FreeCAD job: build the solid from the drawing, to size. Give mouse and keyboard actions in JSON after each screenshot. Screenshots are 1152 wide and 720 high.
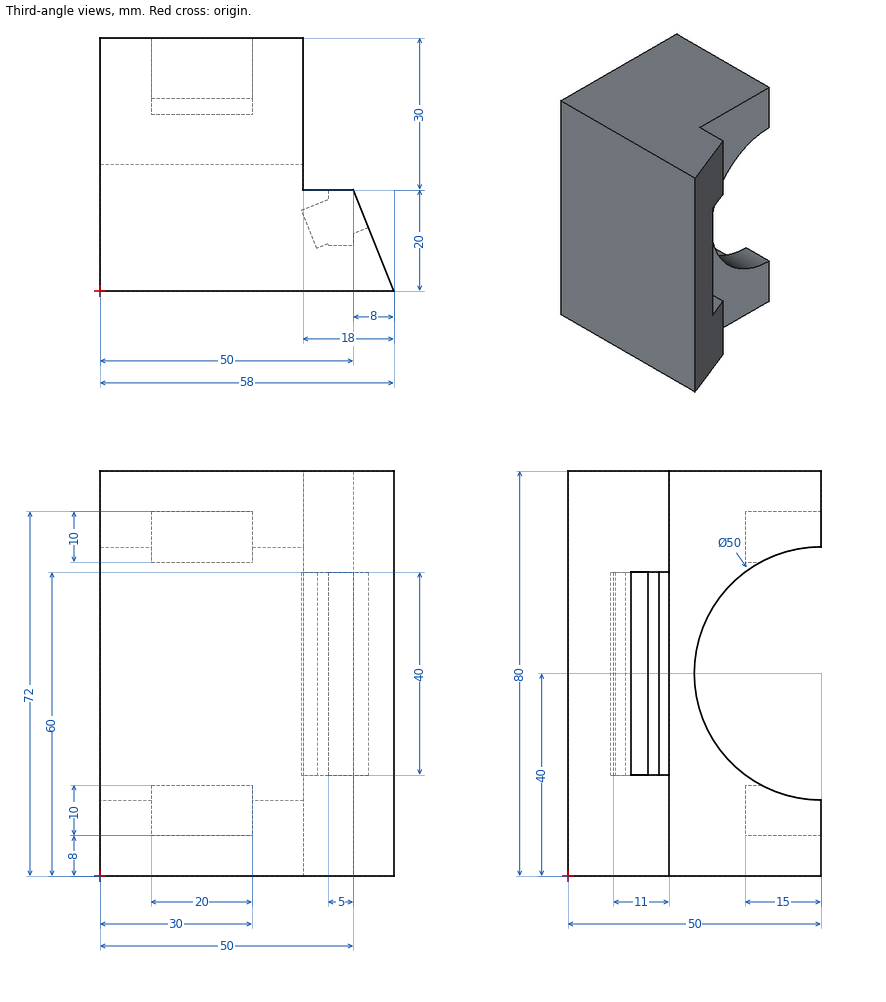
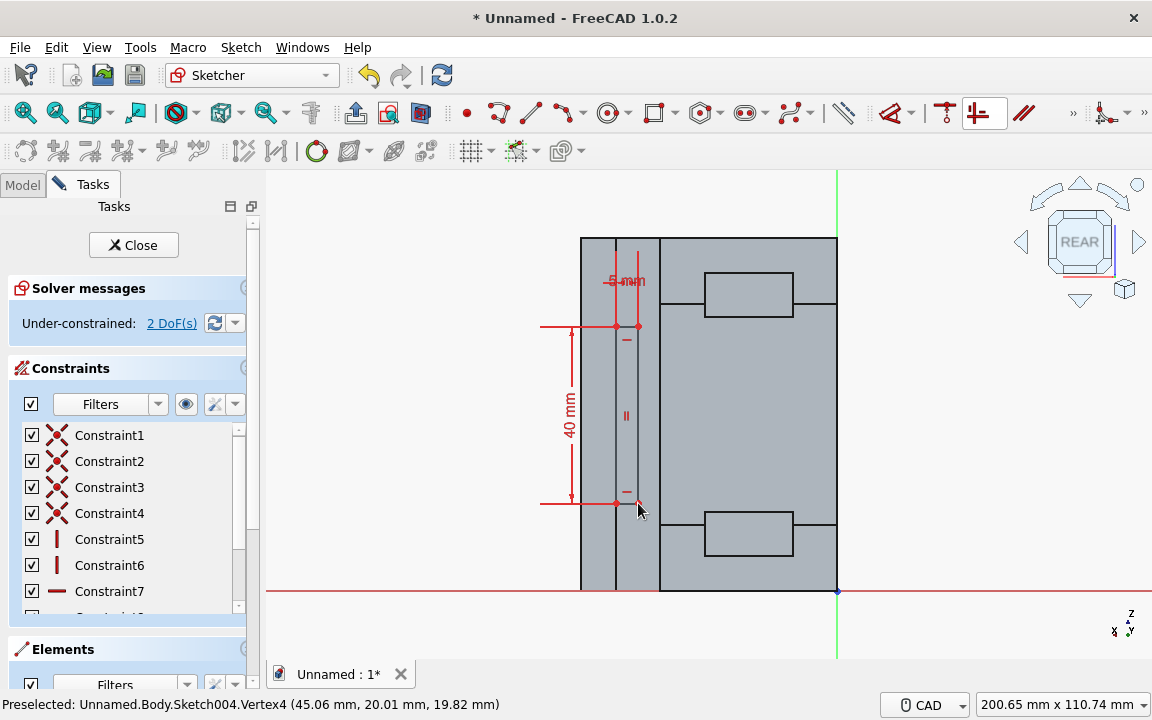
{"action": "left_click", "coordinate": [890, 114]}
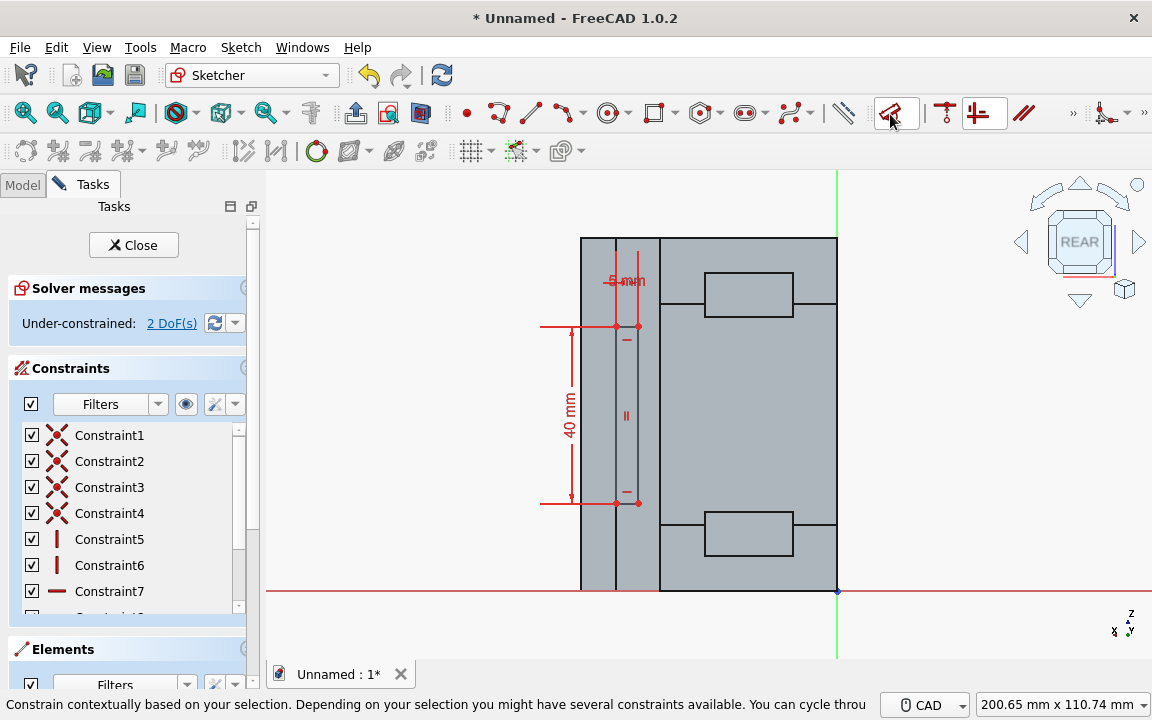
{"action": "left_click", "coordinate": [616, 327]}
{"action": "left_click", "coordinate": [727, 625]}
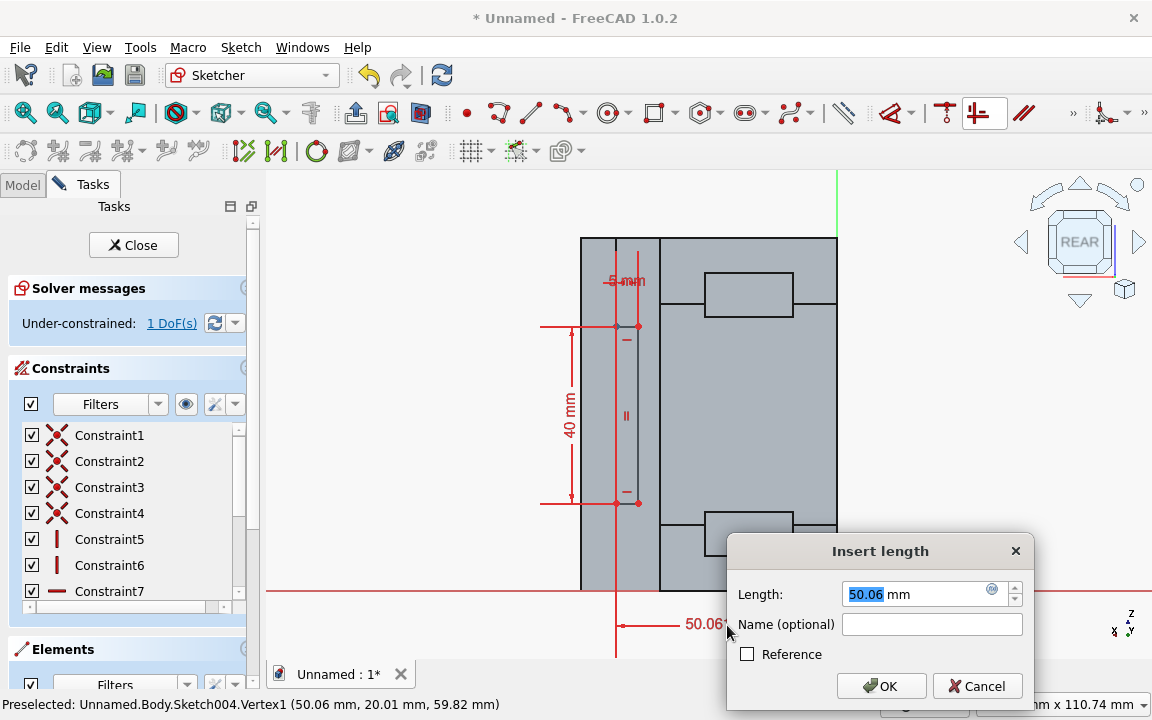
{"action": "type", "text": "50"}
{"action": "key", "text": "Return"}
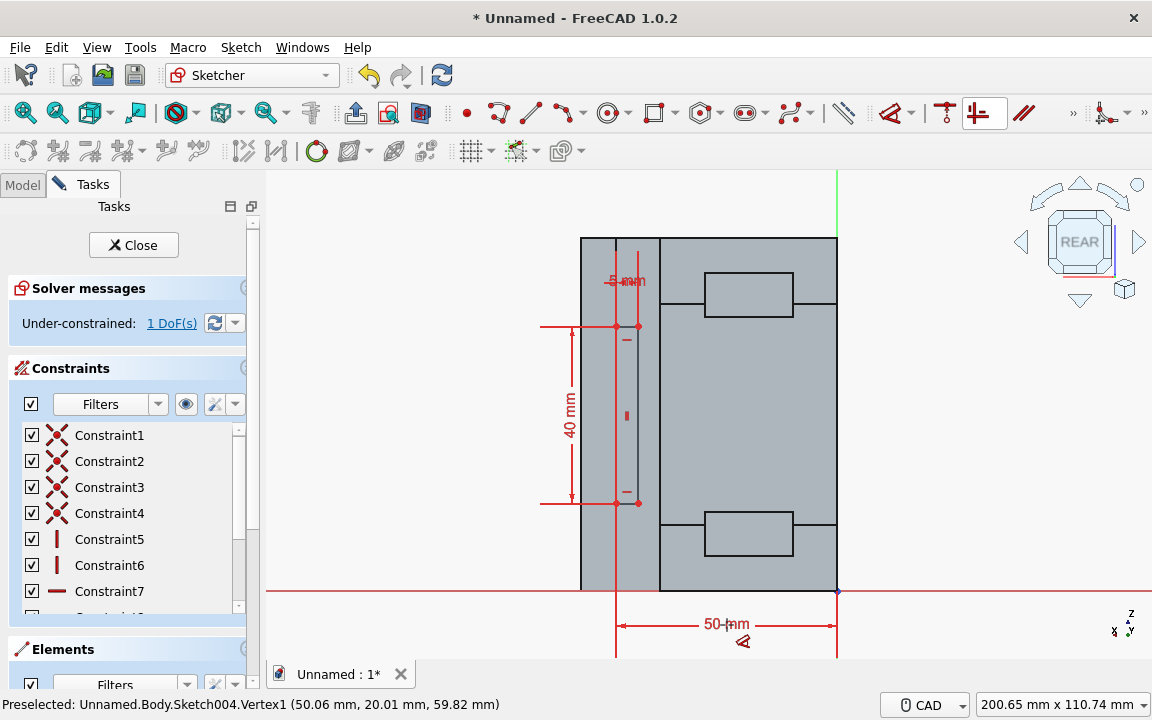
{"action": "left_click", "coordinate": [616, 327]}
{"action": "left_click", "coordinate": [871, 459]}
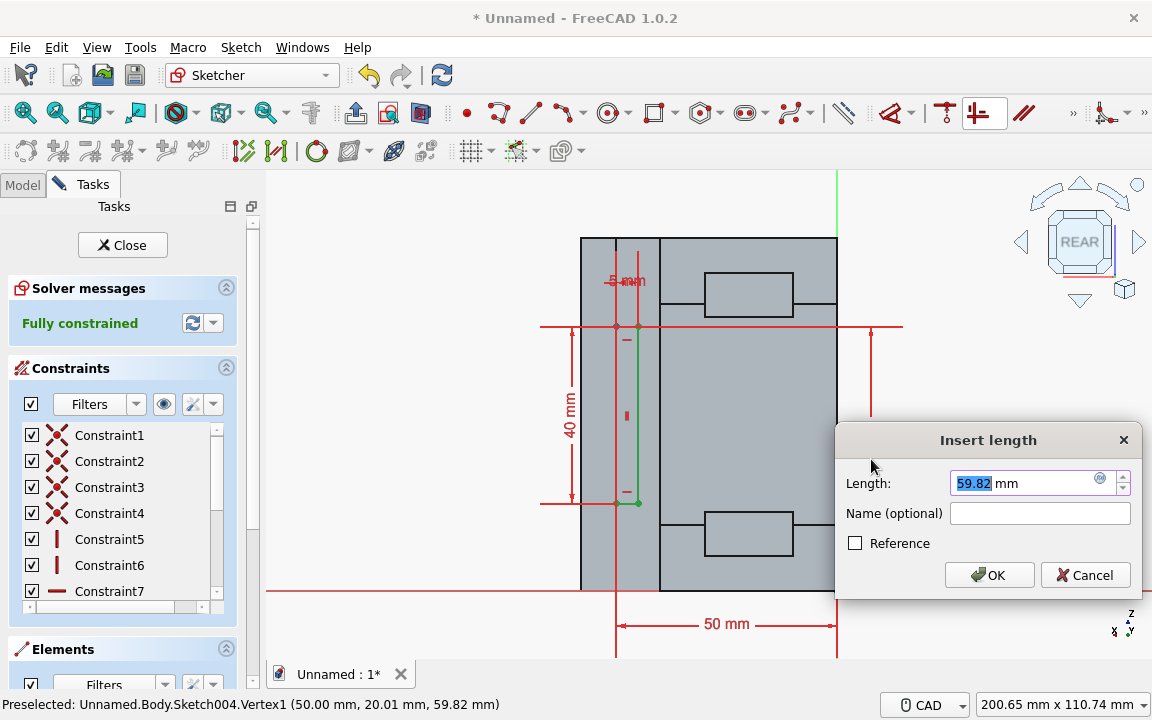
{"action": "type", "text": "60"}
{"action": "key", "text": "Return"}
{"action": "key", "text": "Escape"}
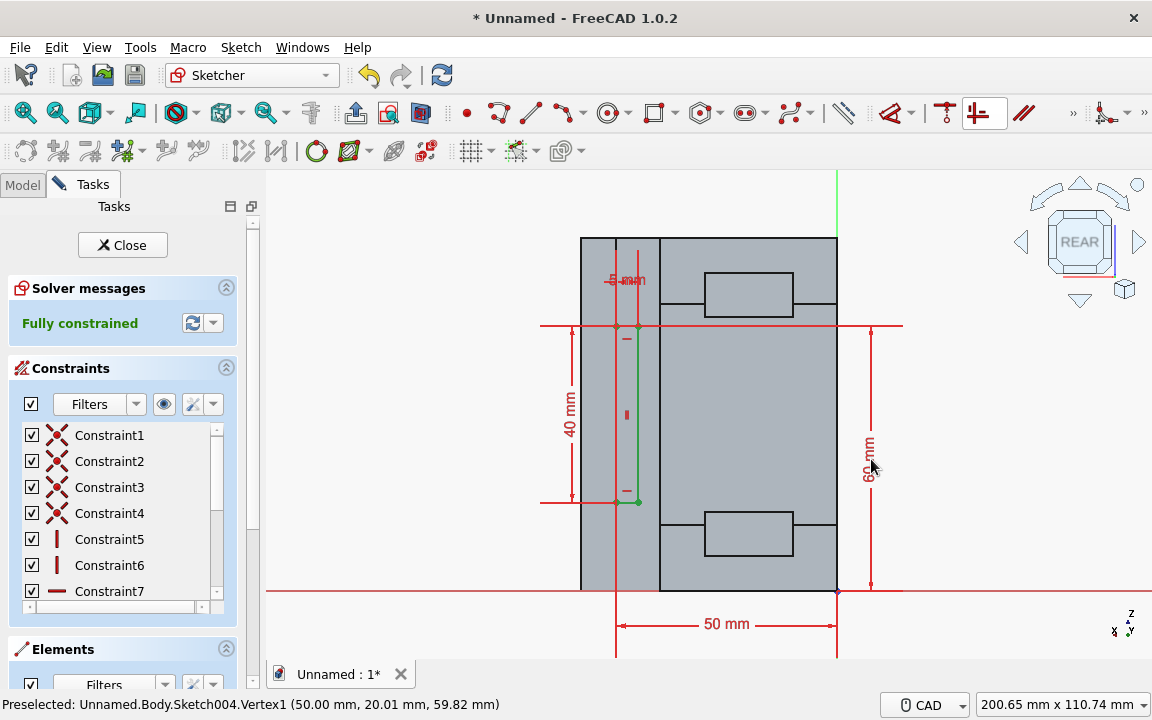
{"action": "left_click", "coordinate": [123, 245]}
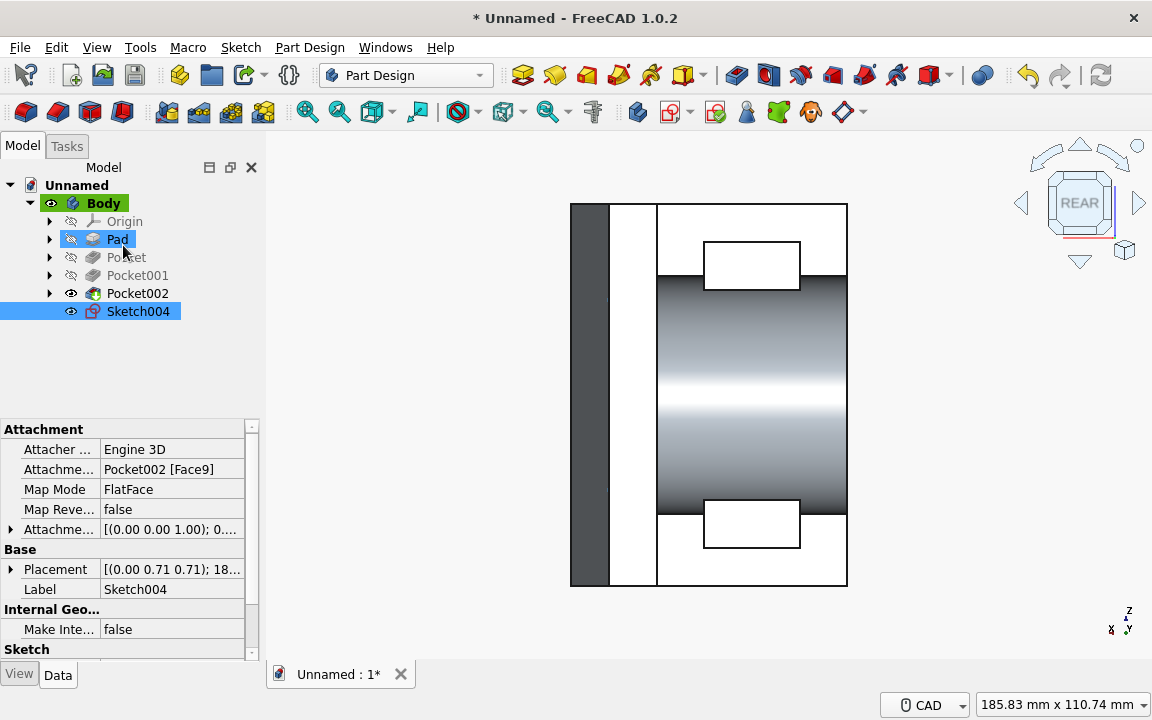
{"action": "left_click", "coordinate": [738, 76]}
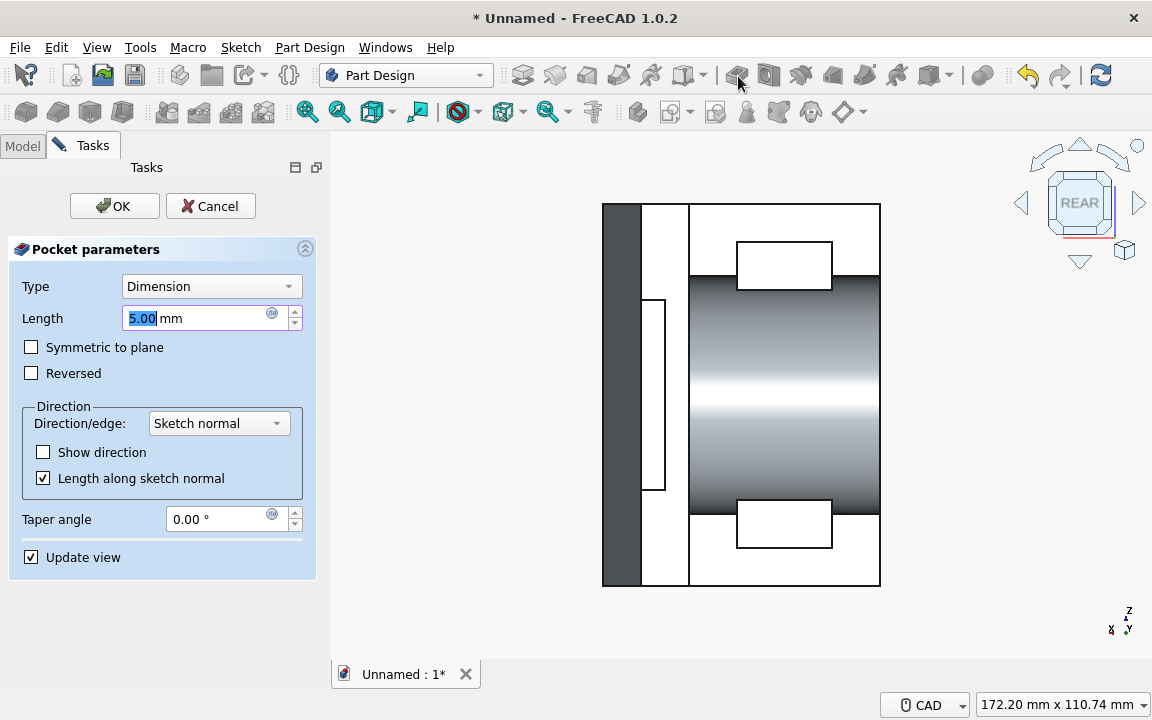
{"action": "type", "text": "11"}
{"action": "key", "text": "Tab"}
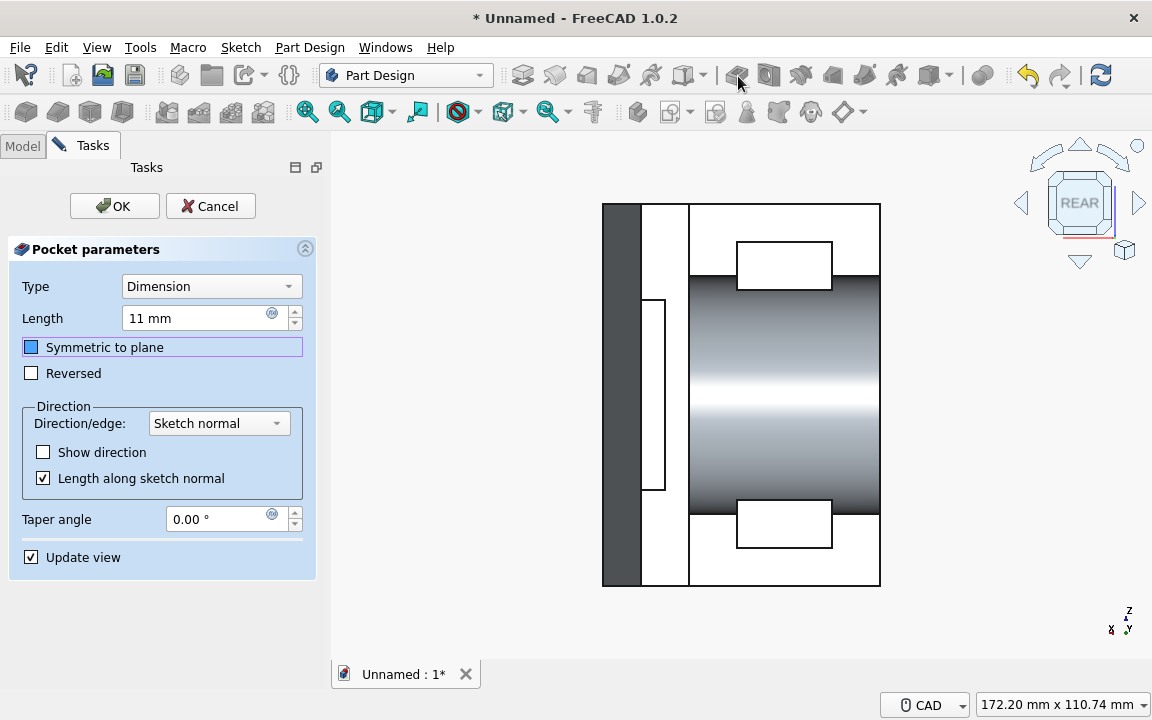
{"action": "left_click", "coordinate": [115, 206]}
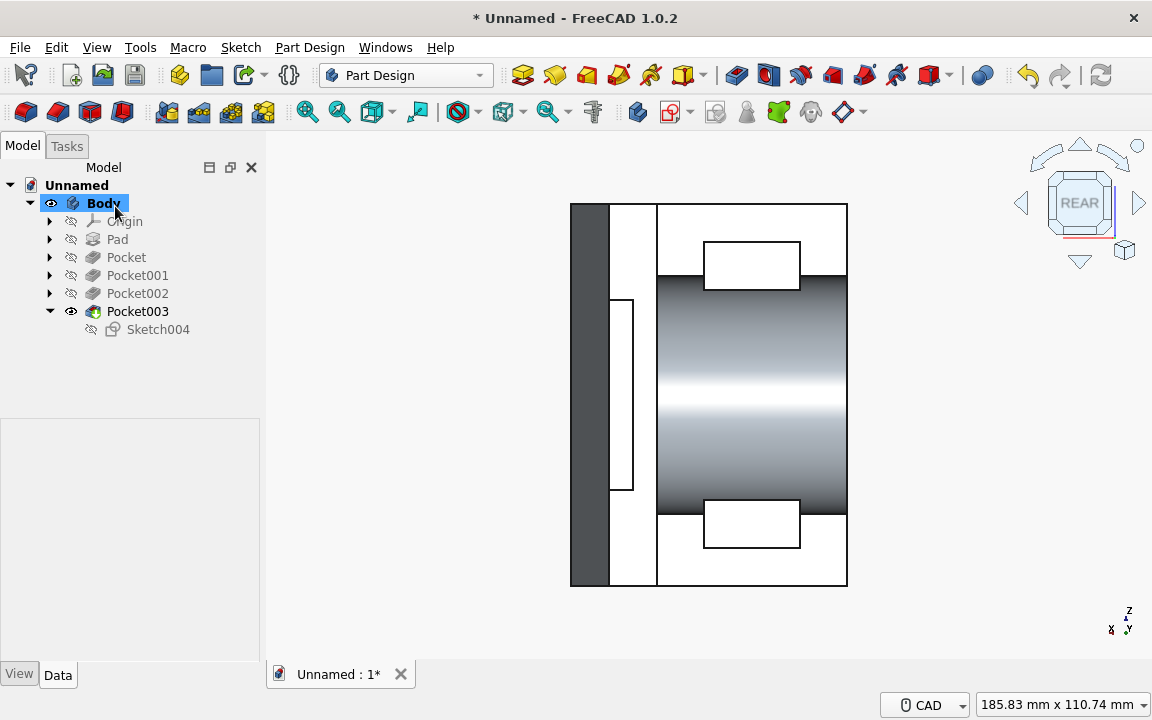
{"action": "left_click", "coordinate": [590, 285]}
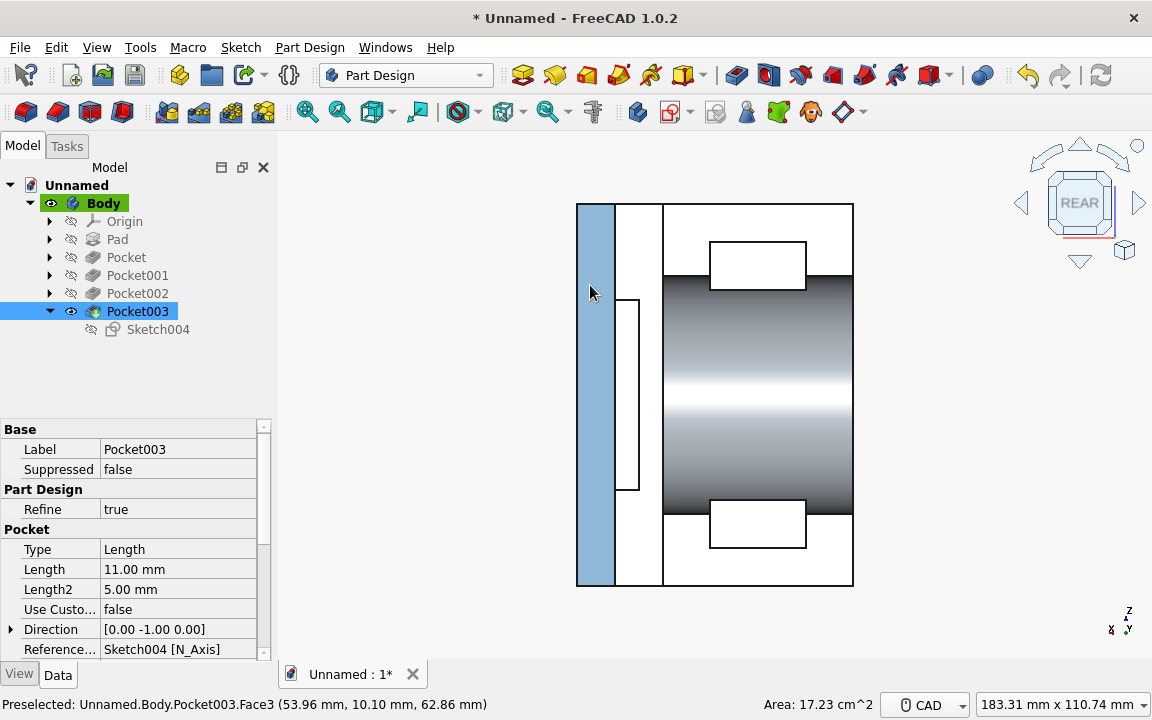
{"action": "left_click", "coordinate": [670, 112]}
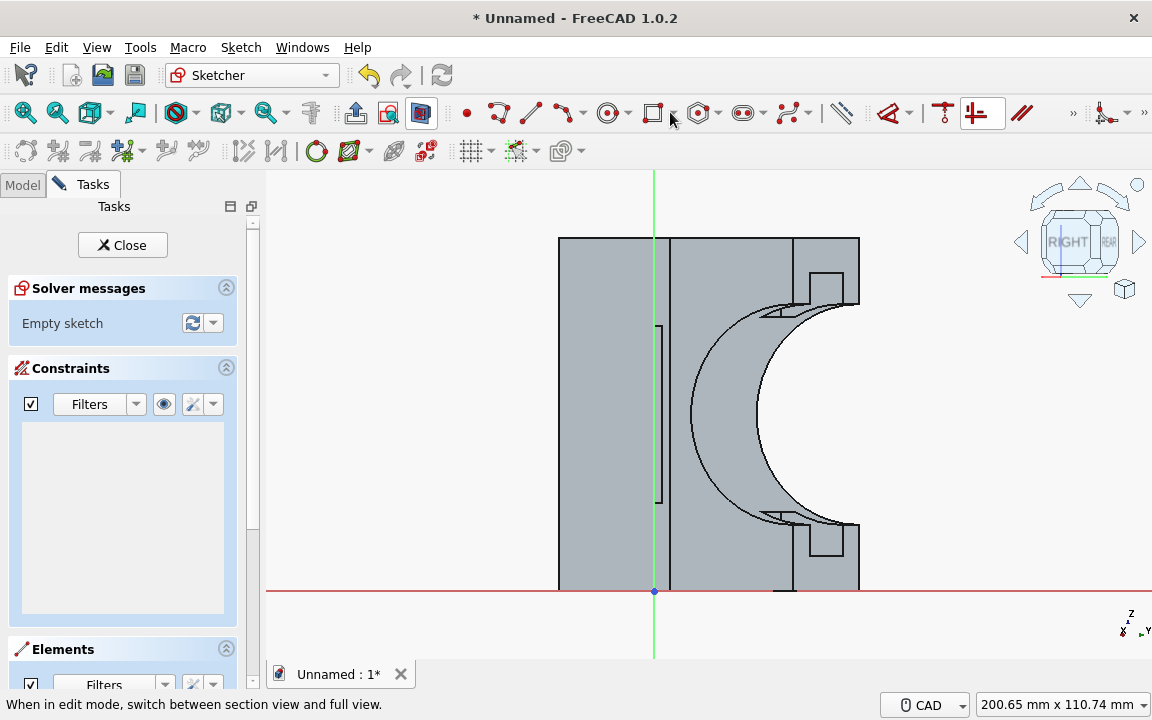
{"action": "left_click", "coordinate": [654, 114]}